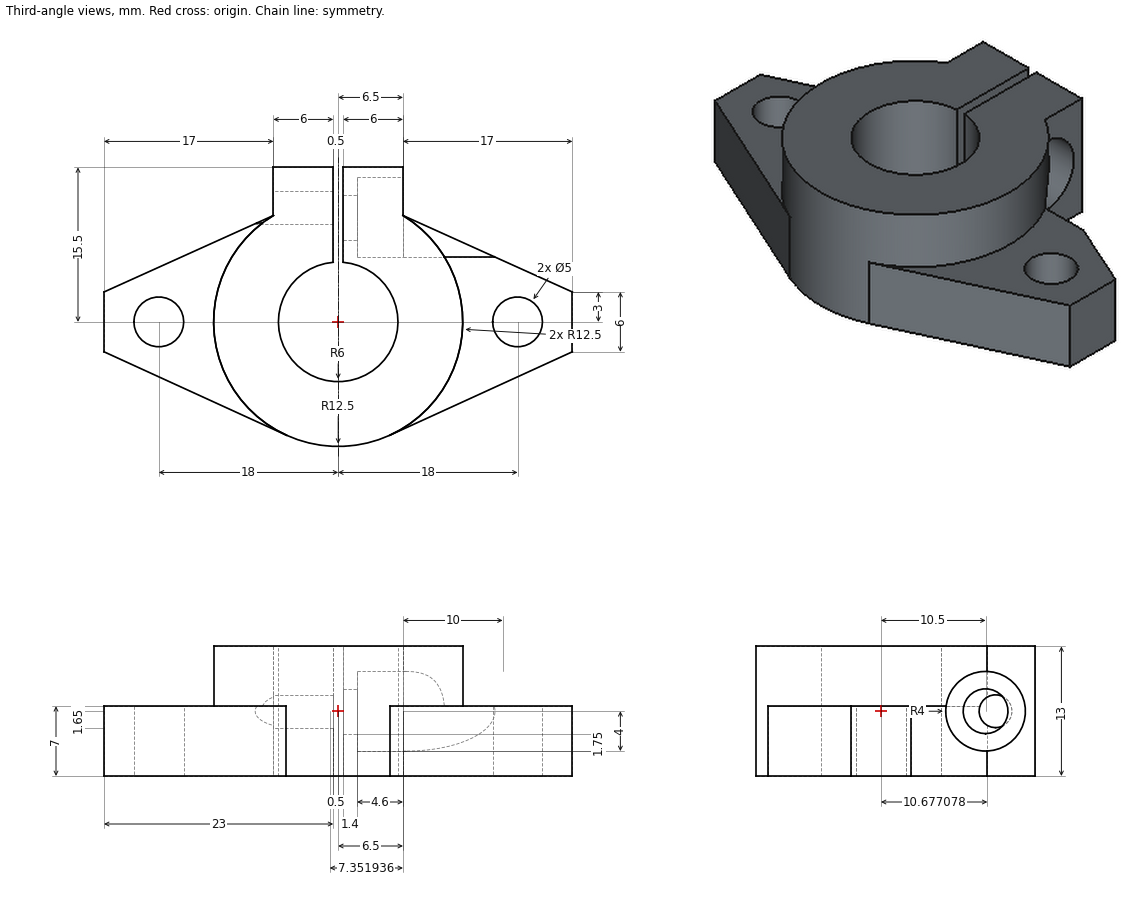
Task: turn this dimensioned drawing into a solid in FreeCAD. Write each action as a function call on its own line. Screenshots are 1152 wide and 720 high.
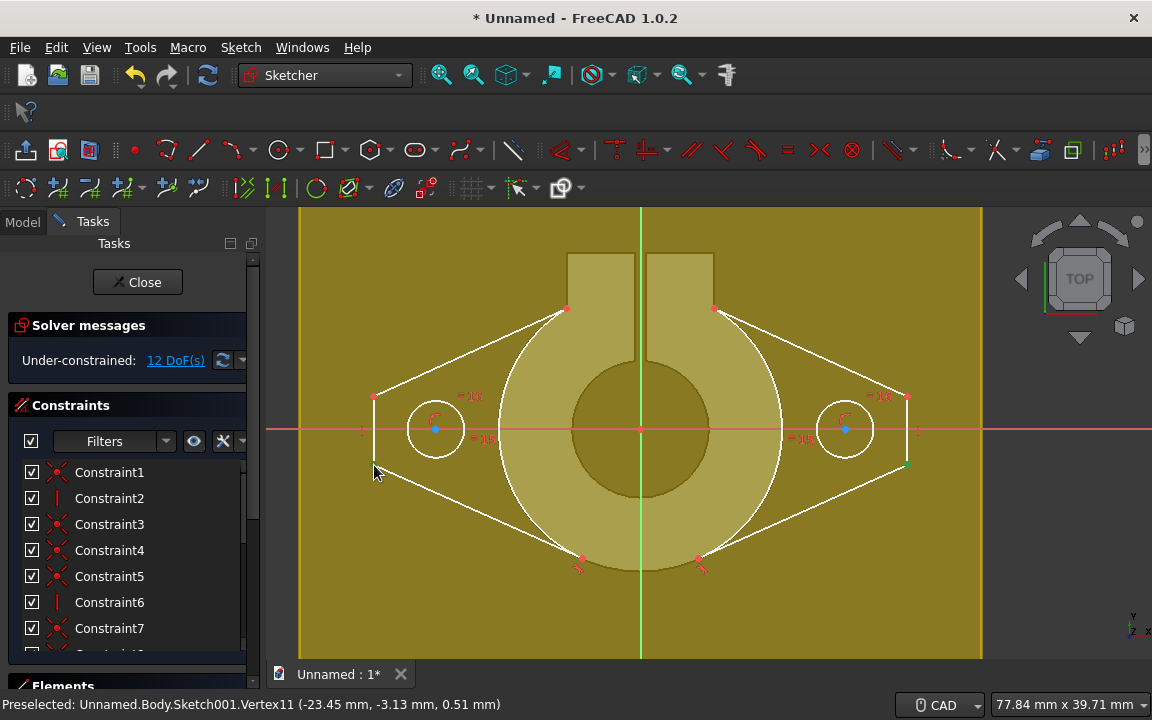
click(641, 603)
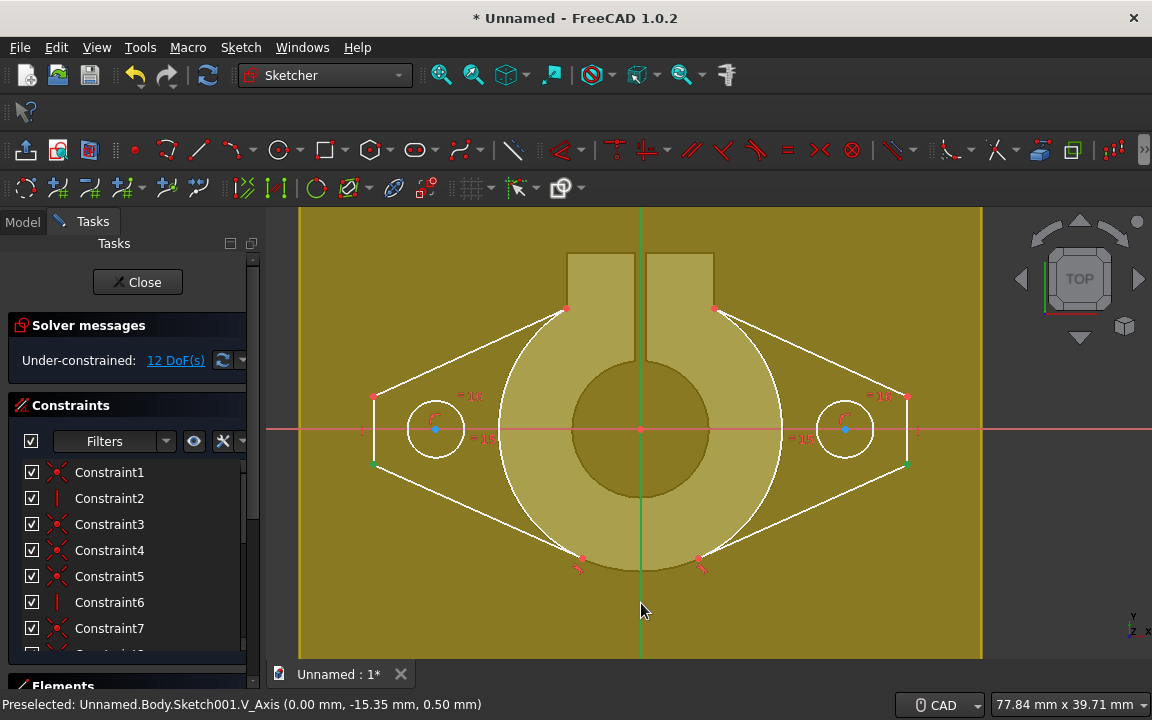
click(820, 150)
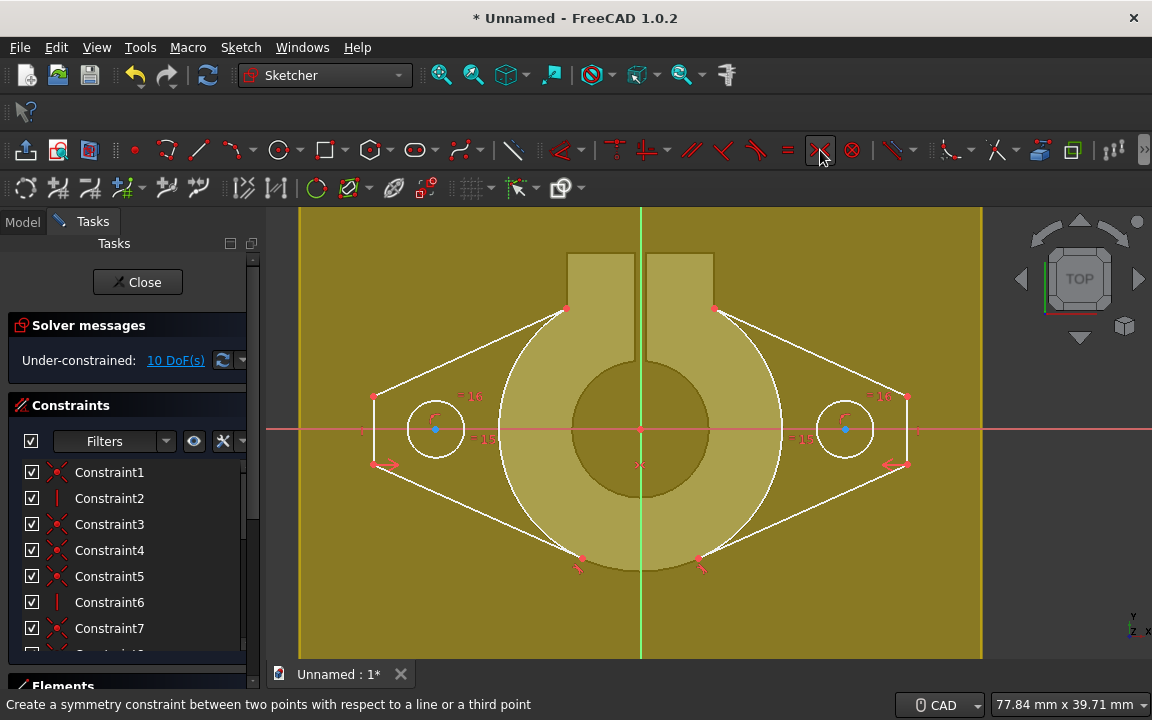
click(560, 150)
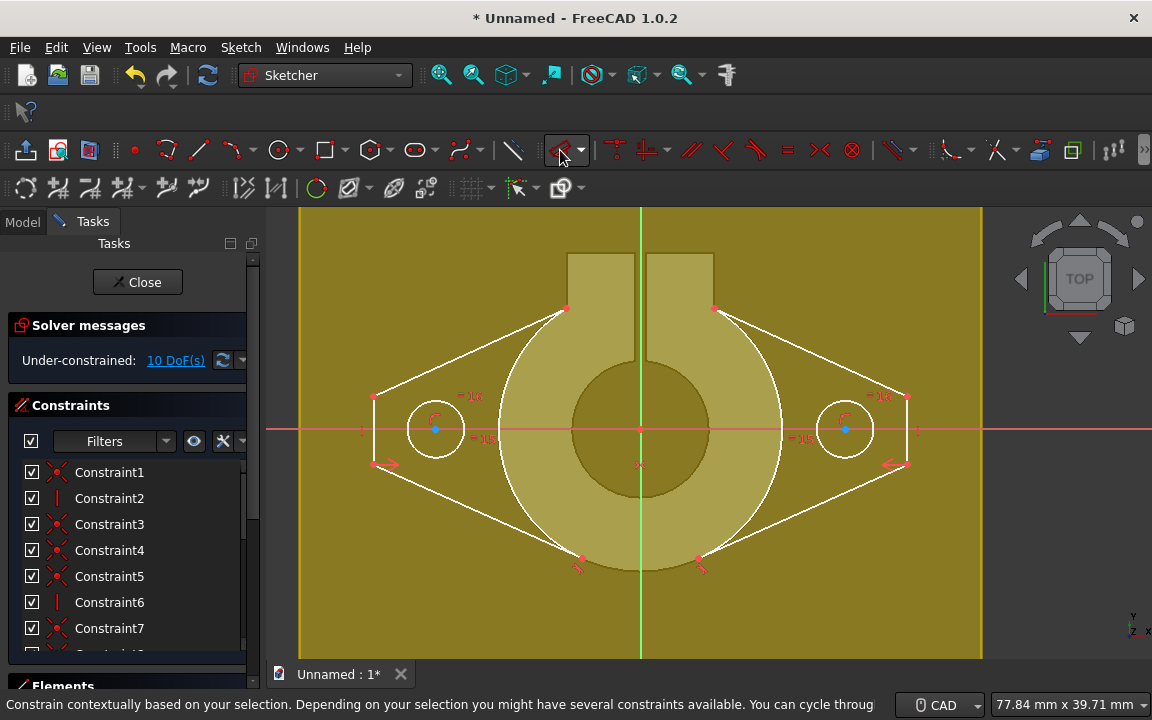
click(765, 497)
click(735, 575)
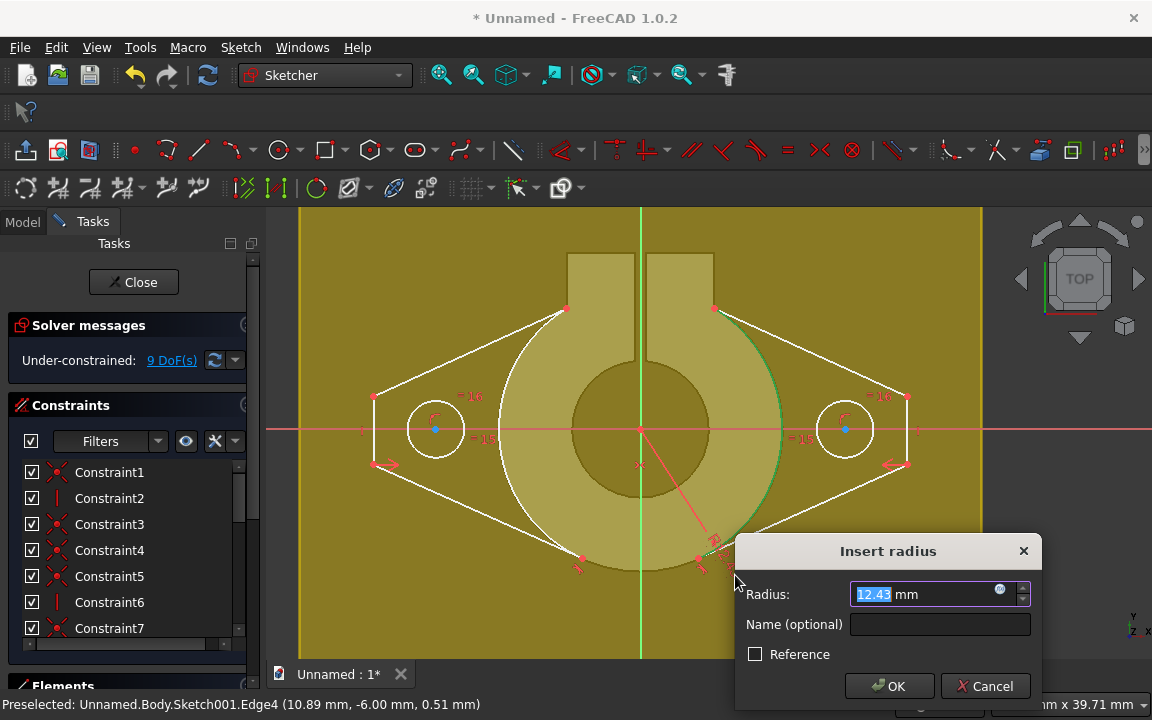
text(12.5)
key(Return)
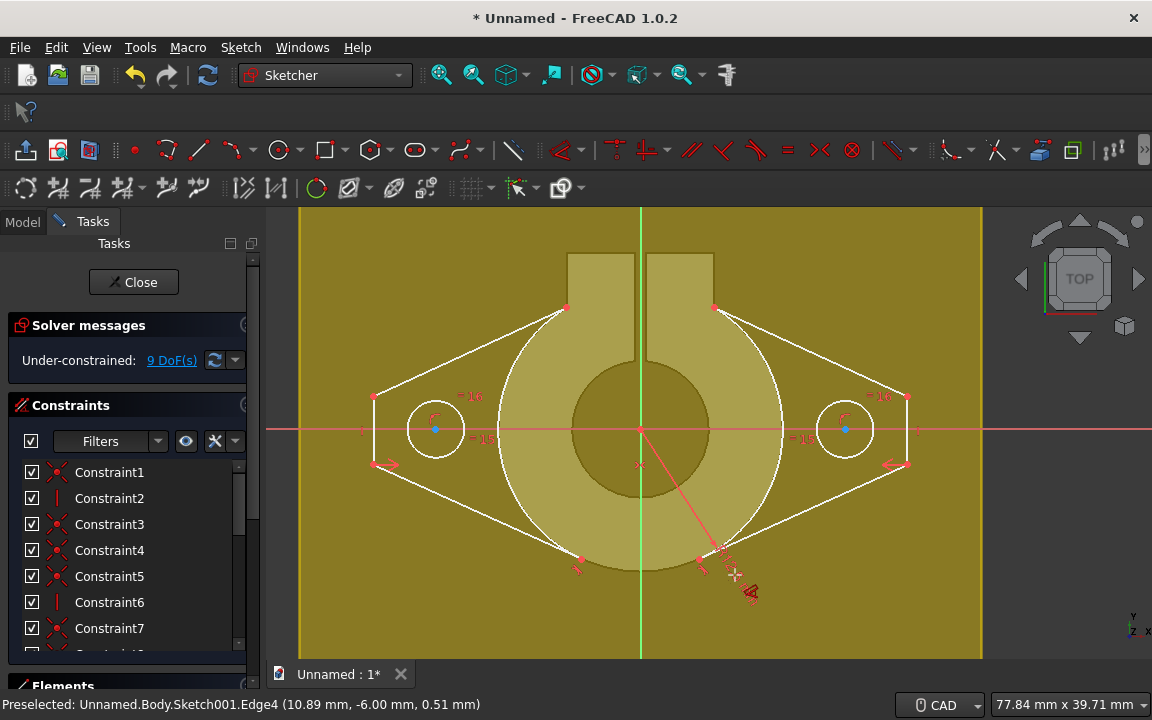
click(865, 409)
click(802, 387)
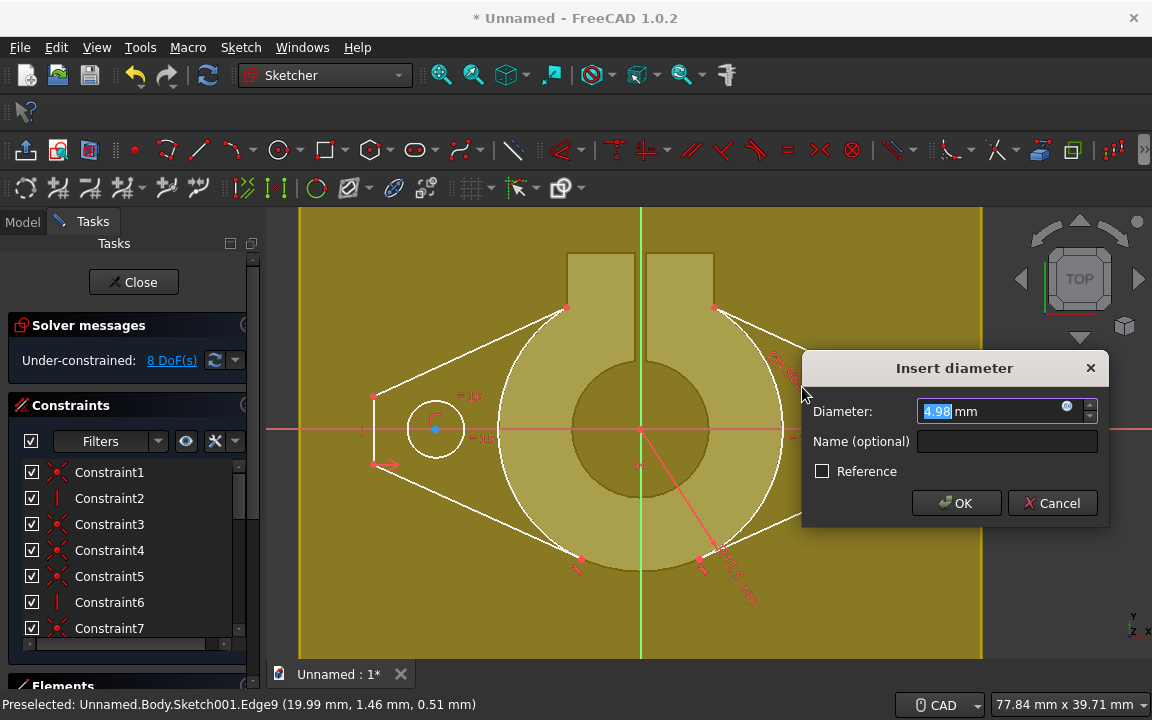
text(5)
key(Return)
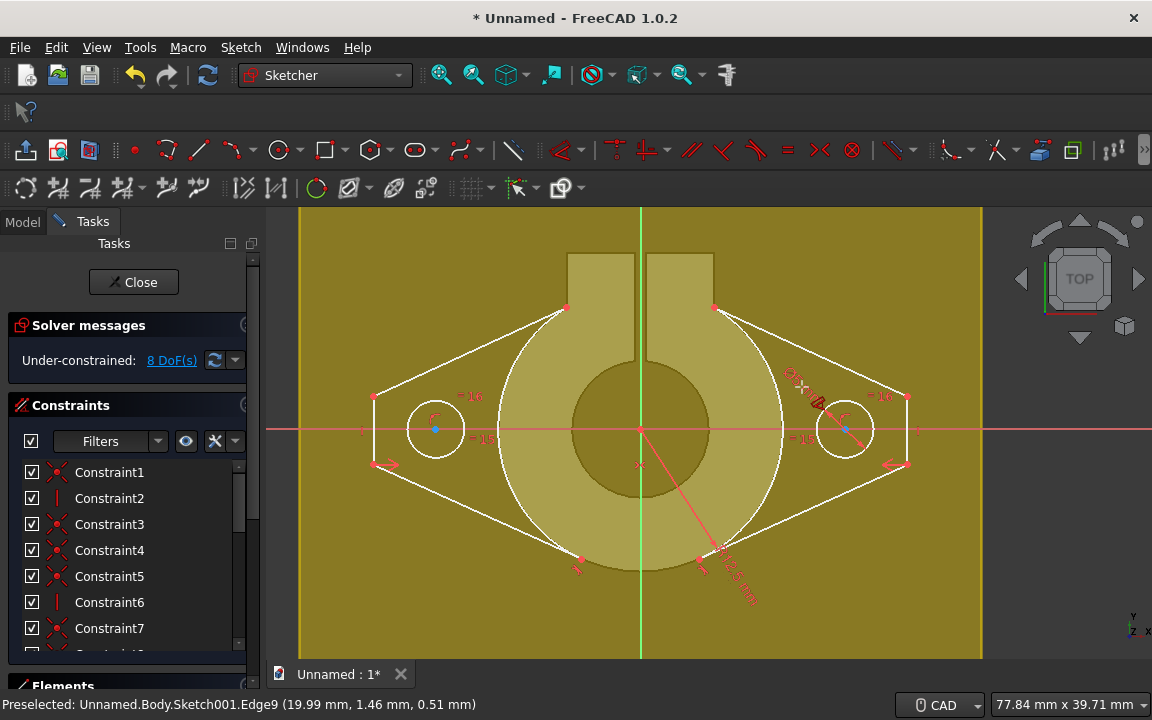
click(907, 417)
click(941, 415)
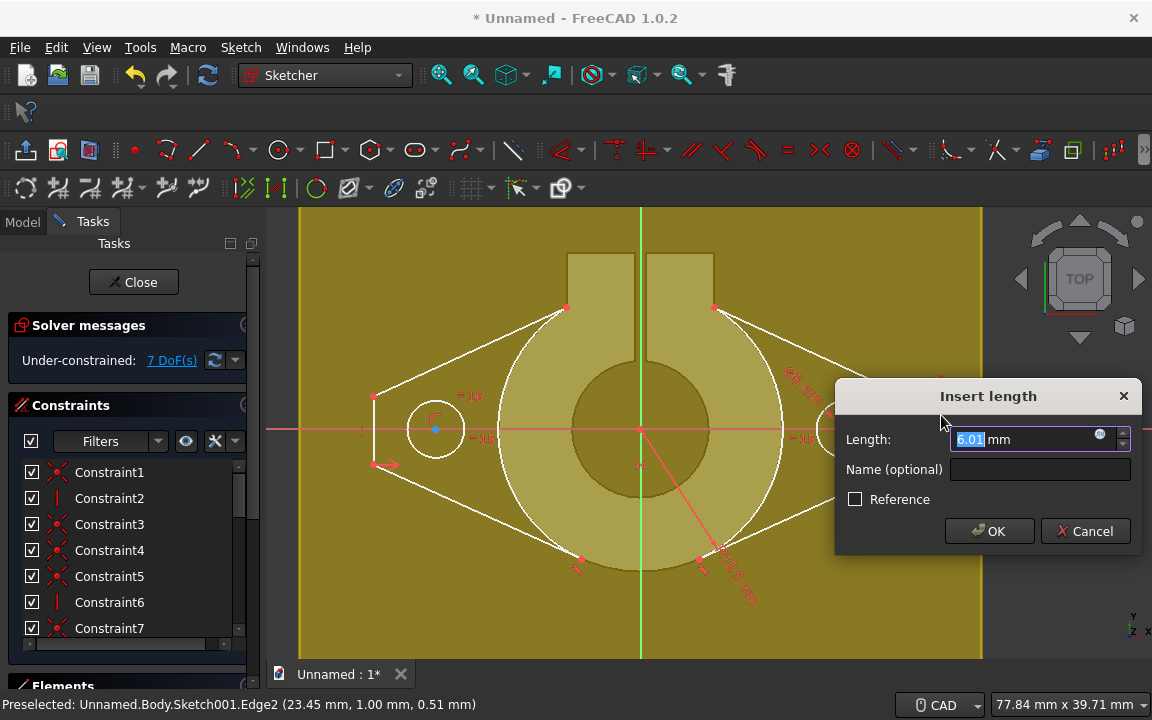
text(6)
key(Return)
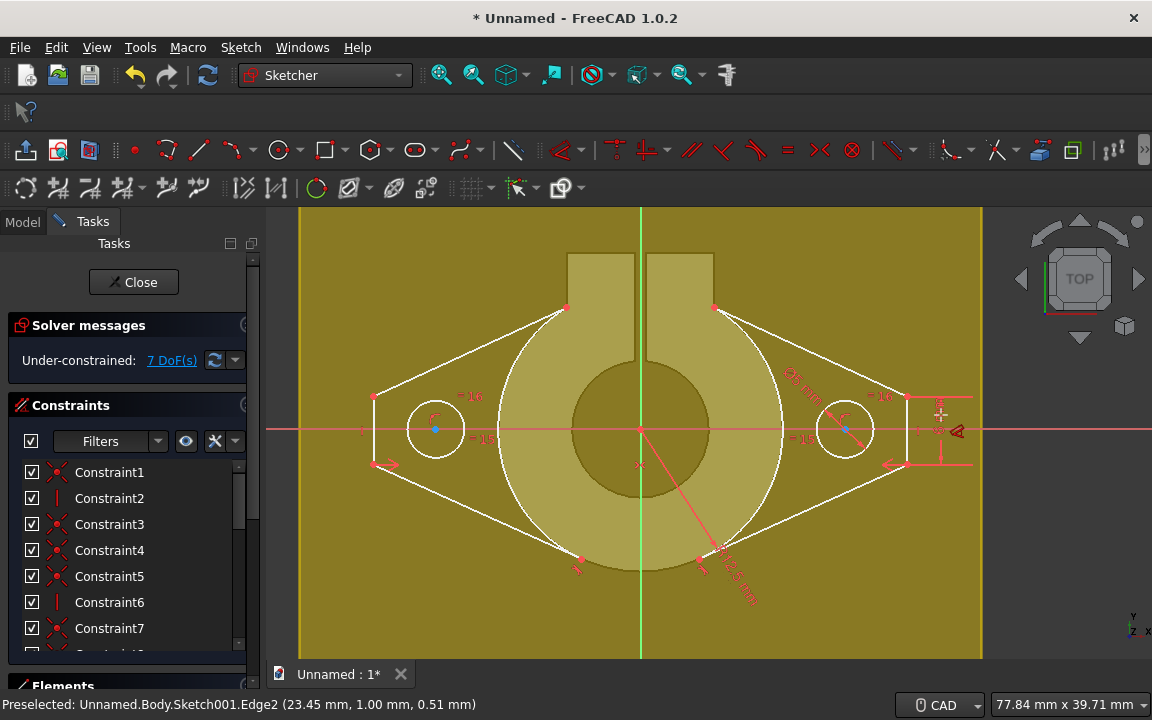
click(374, 444)
click(340, 415)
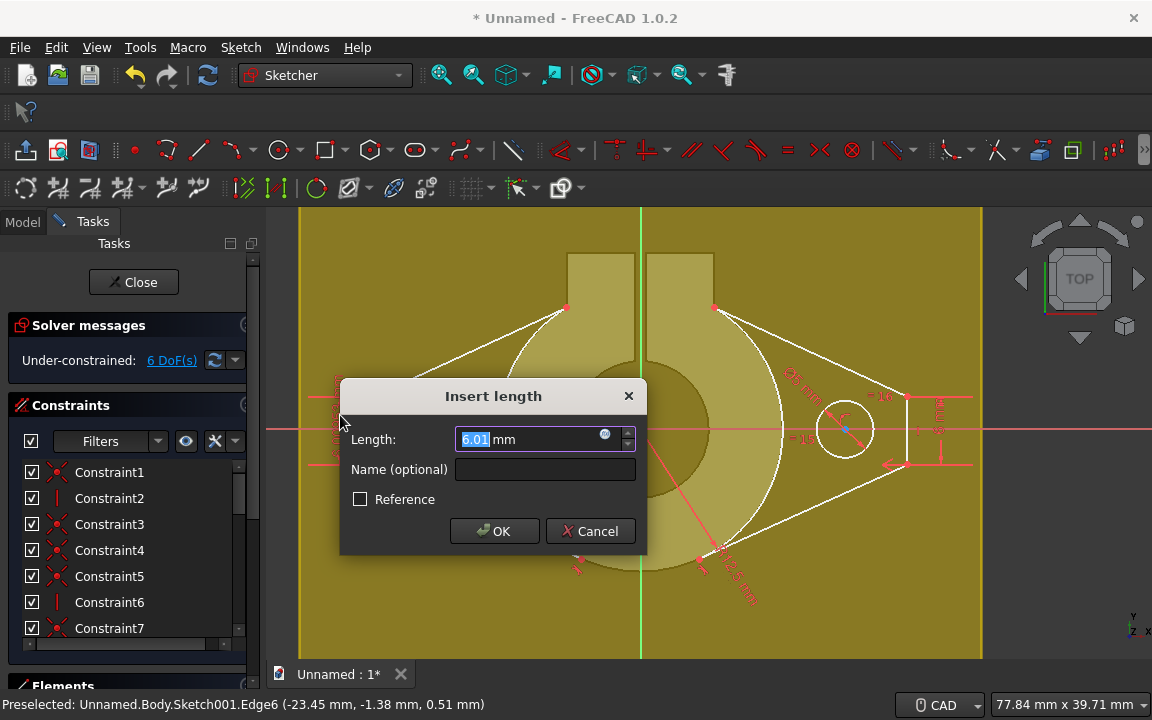
text(6)
key(Return)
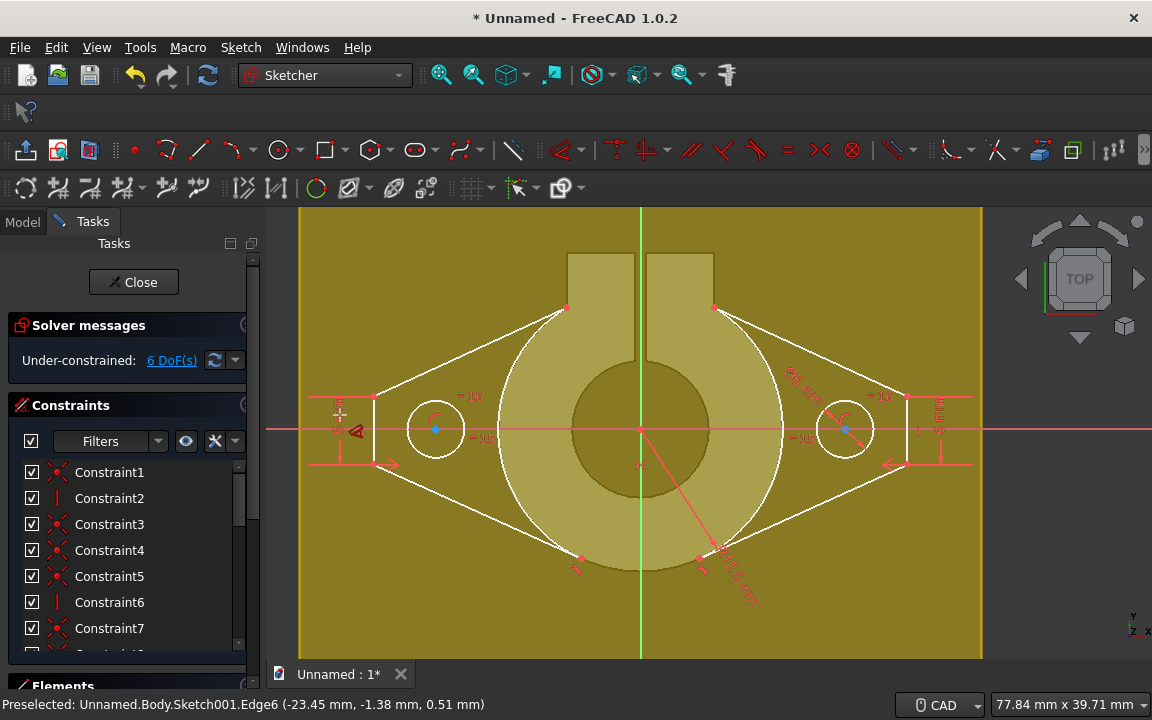
click(907, 397)
click(607, 413)